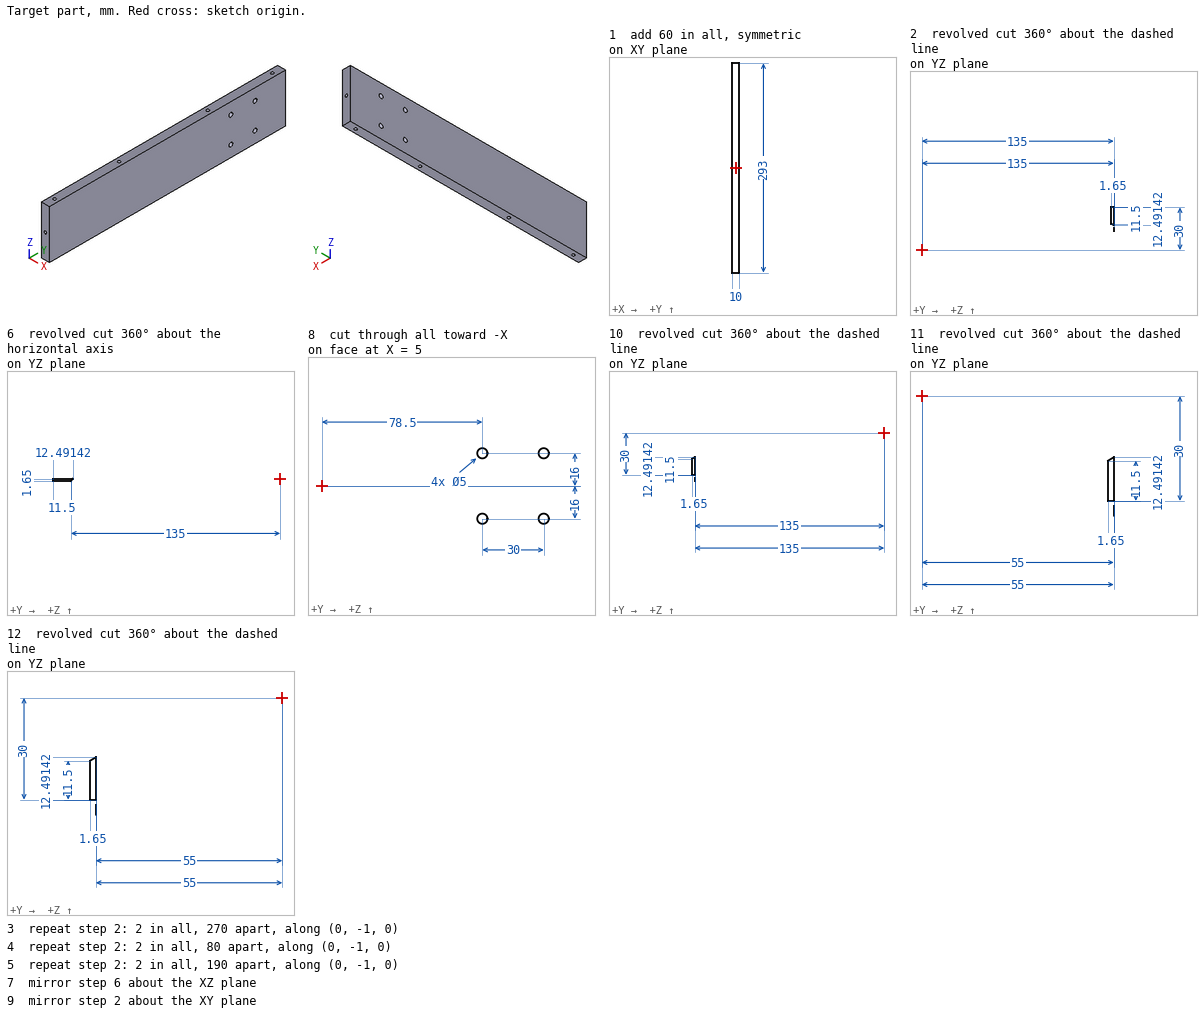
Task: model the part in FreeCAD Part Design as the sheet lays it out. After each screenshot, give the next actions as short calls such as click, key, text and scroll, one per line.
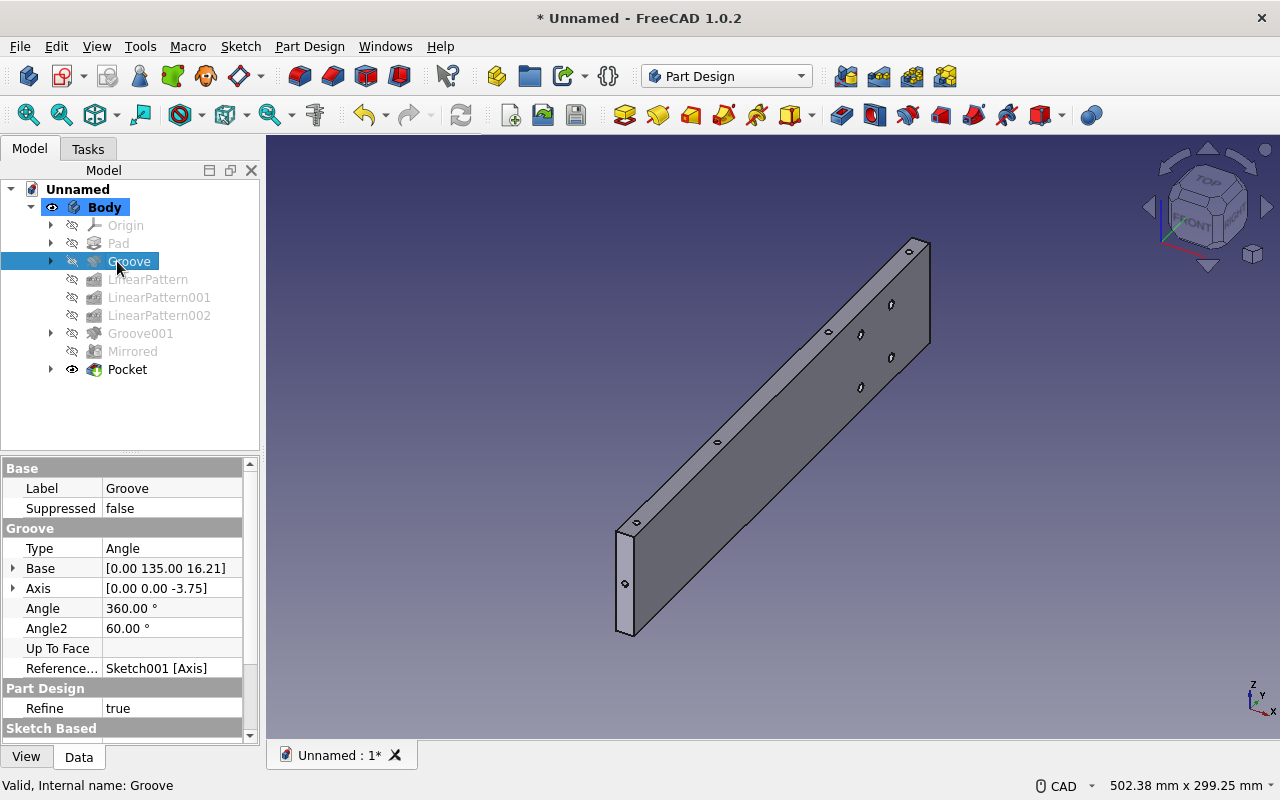
click(846, 76)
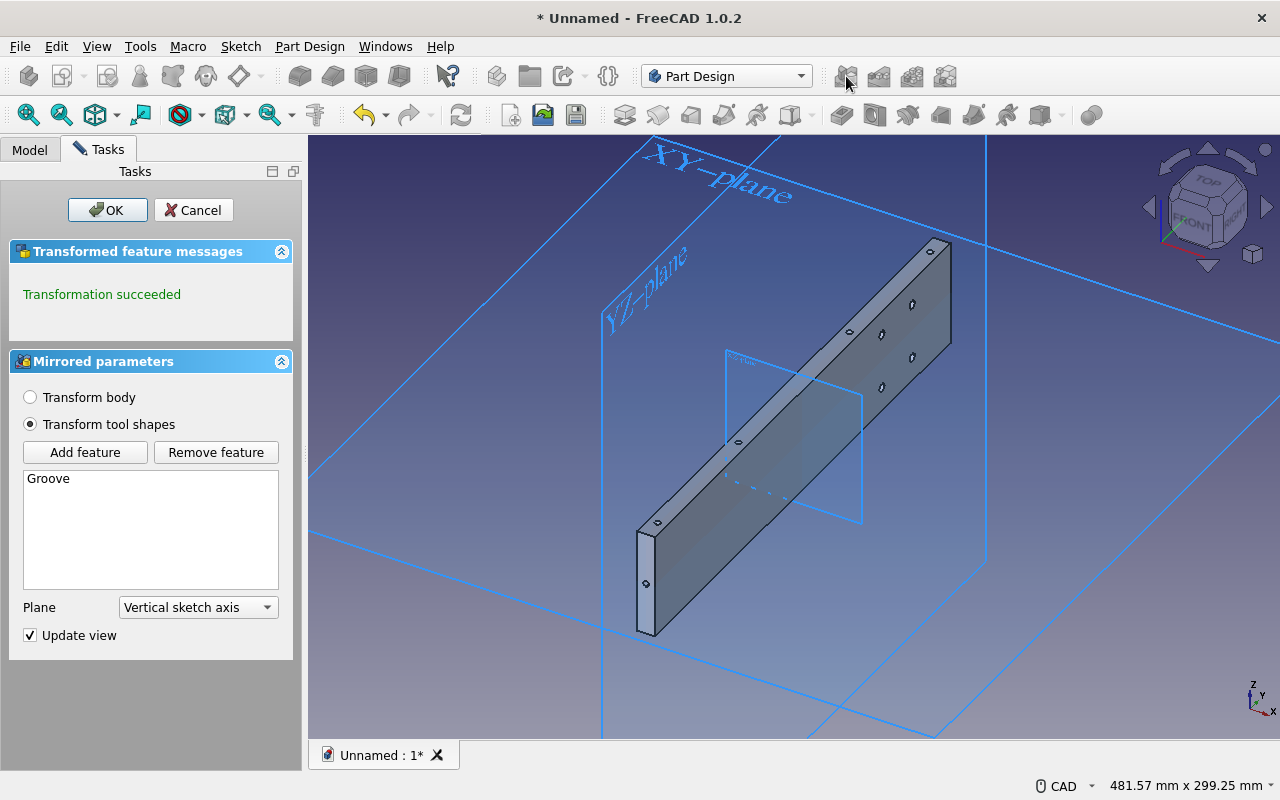
click(199, 608)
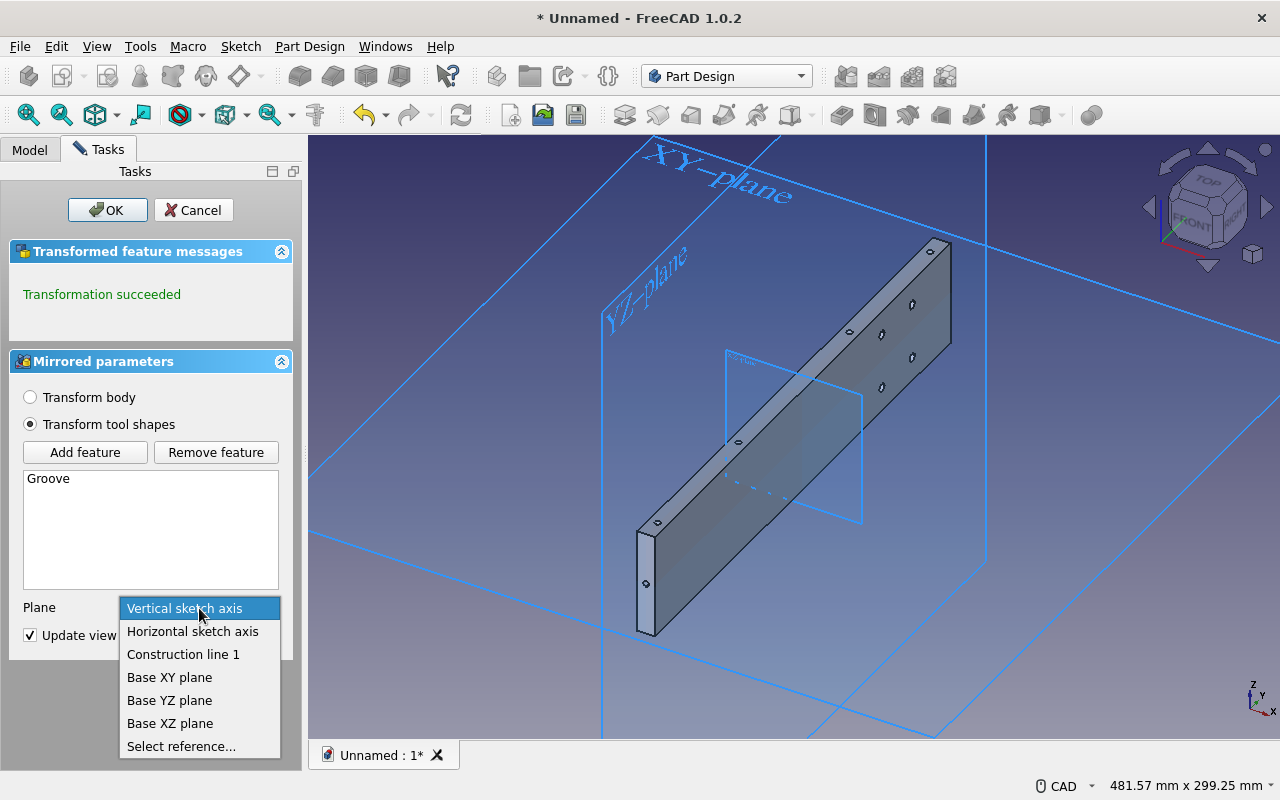
click(198, 678)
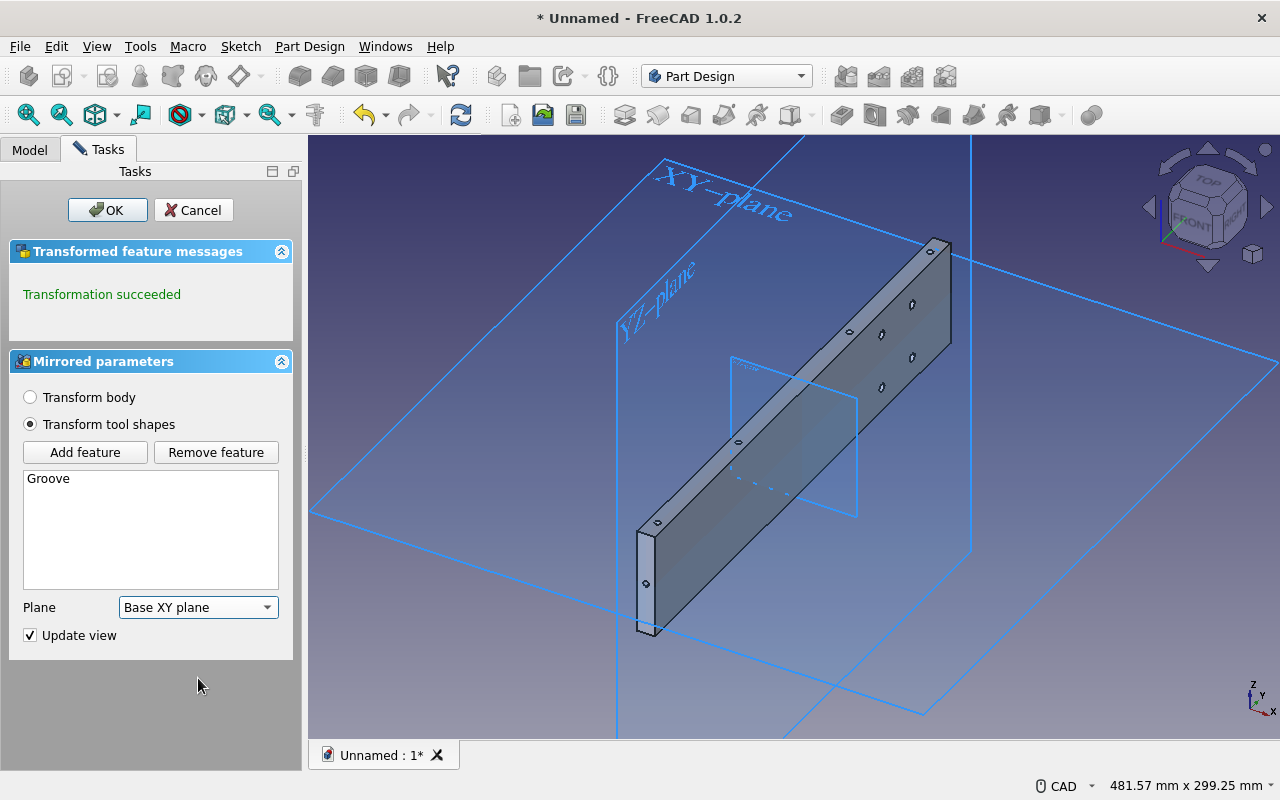
click(108, 210)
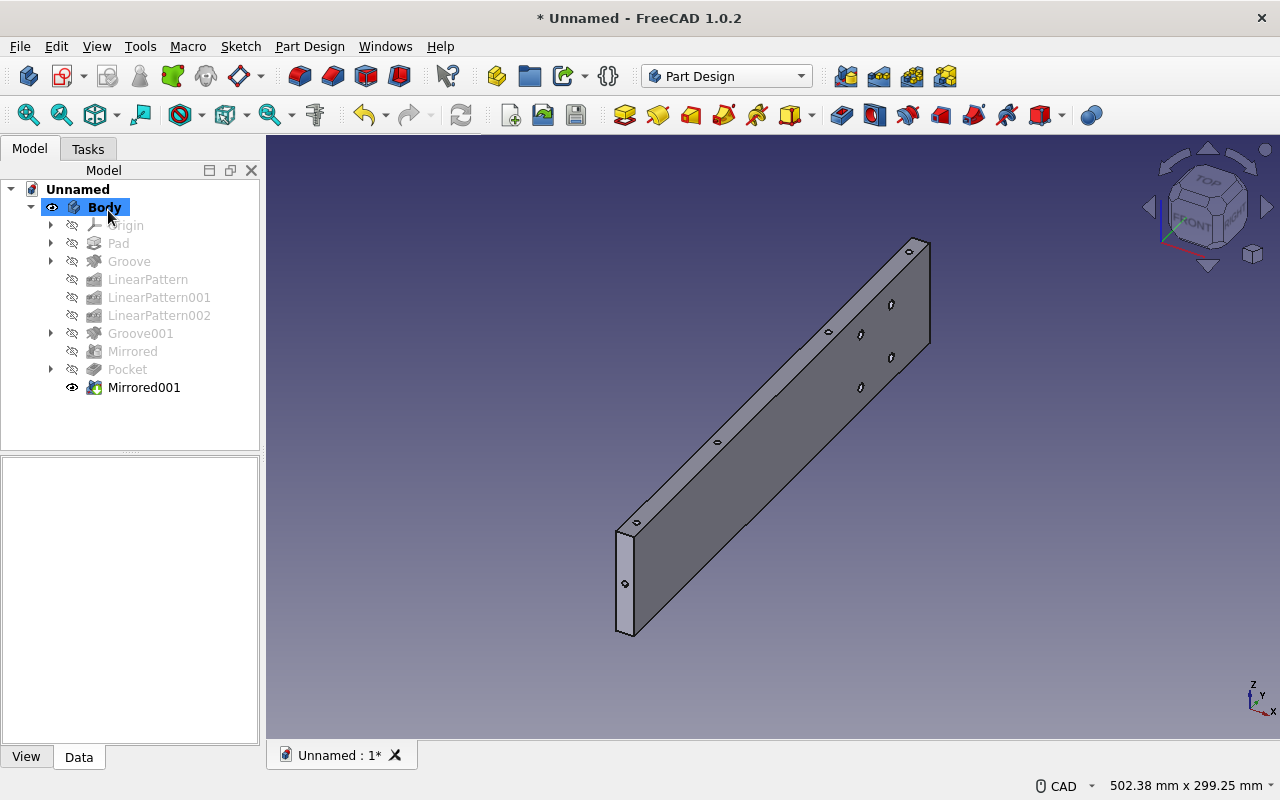
click(62, 76)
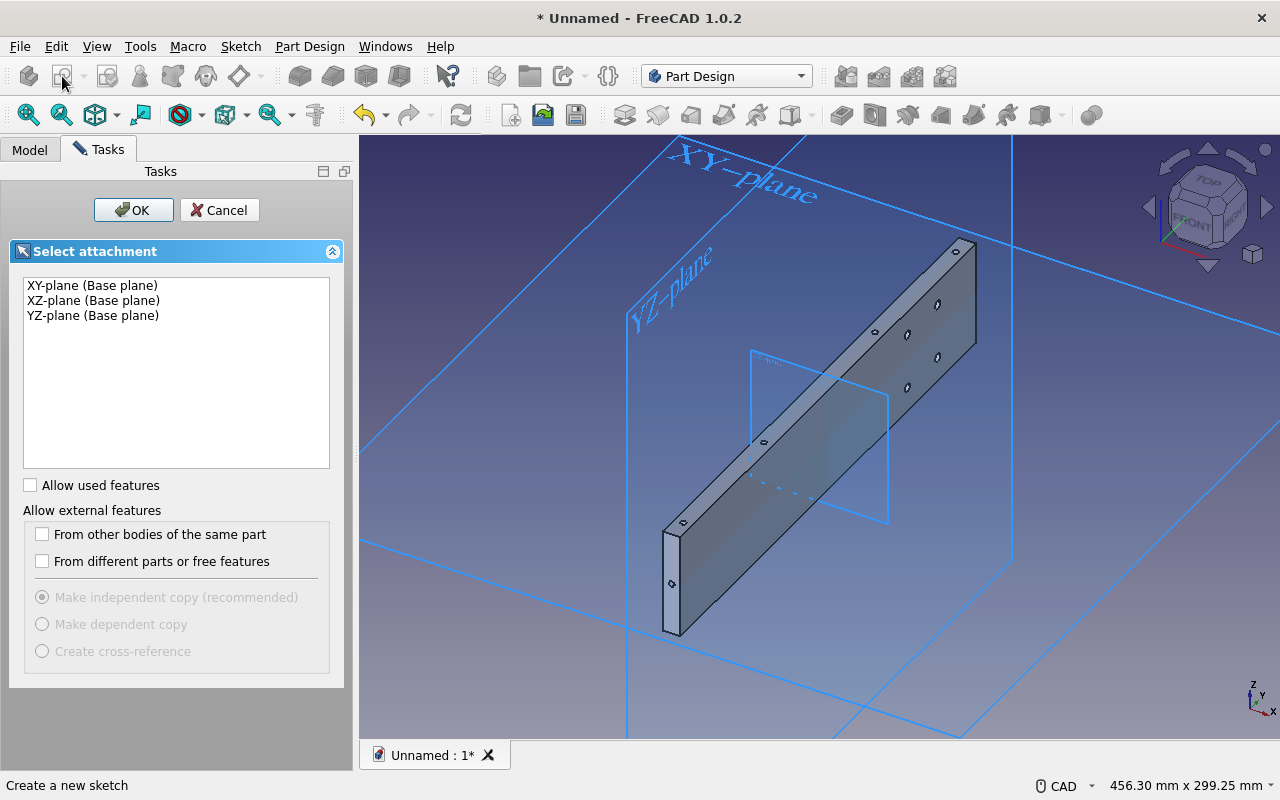
click(84, 316)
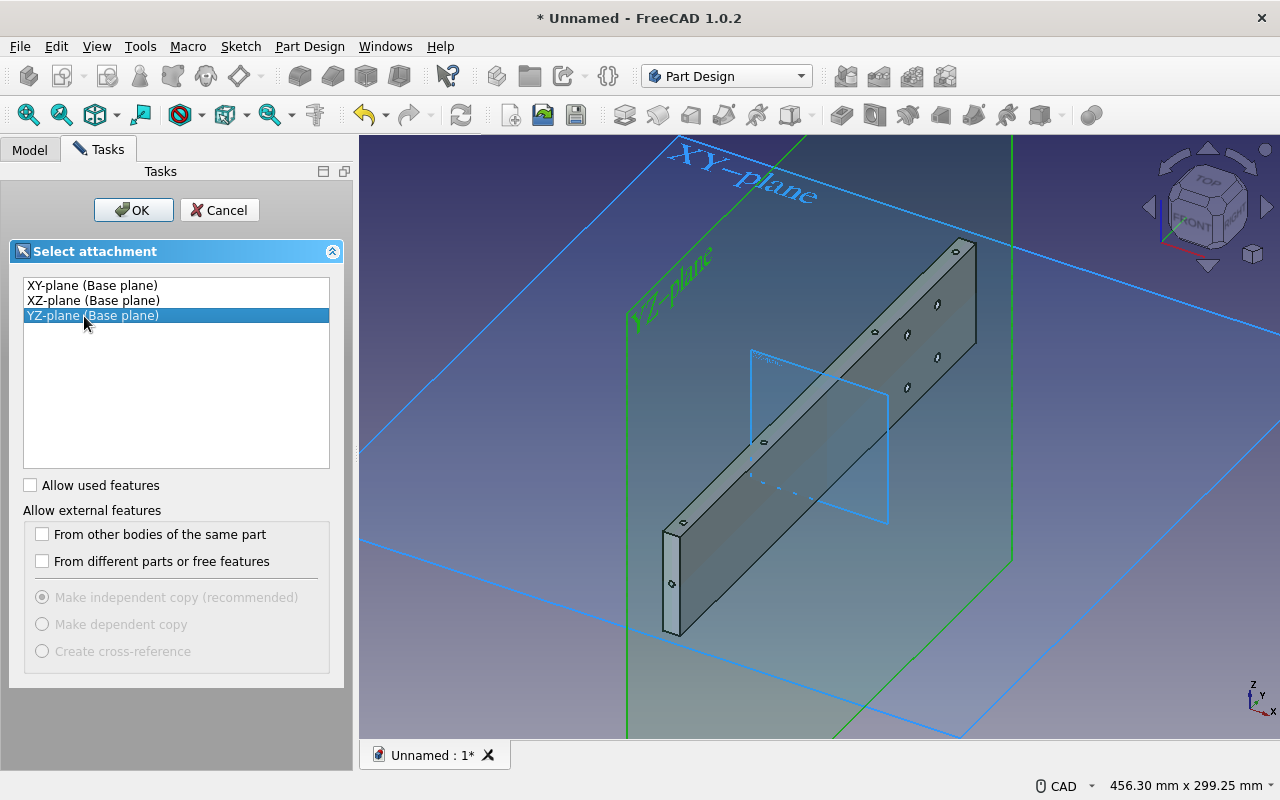
click(134, 210)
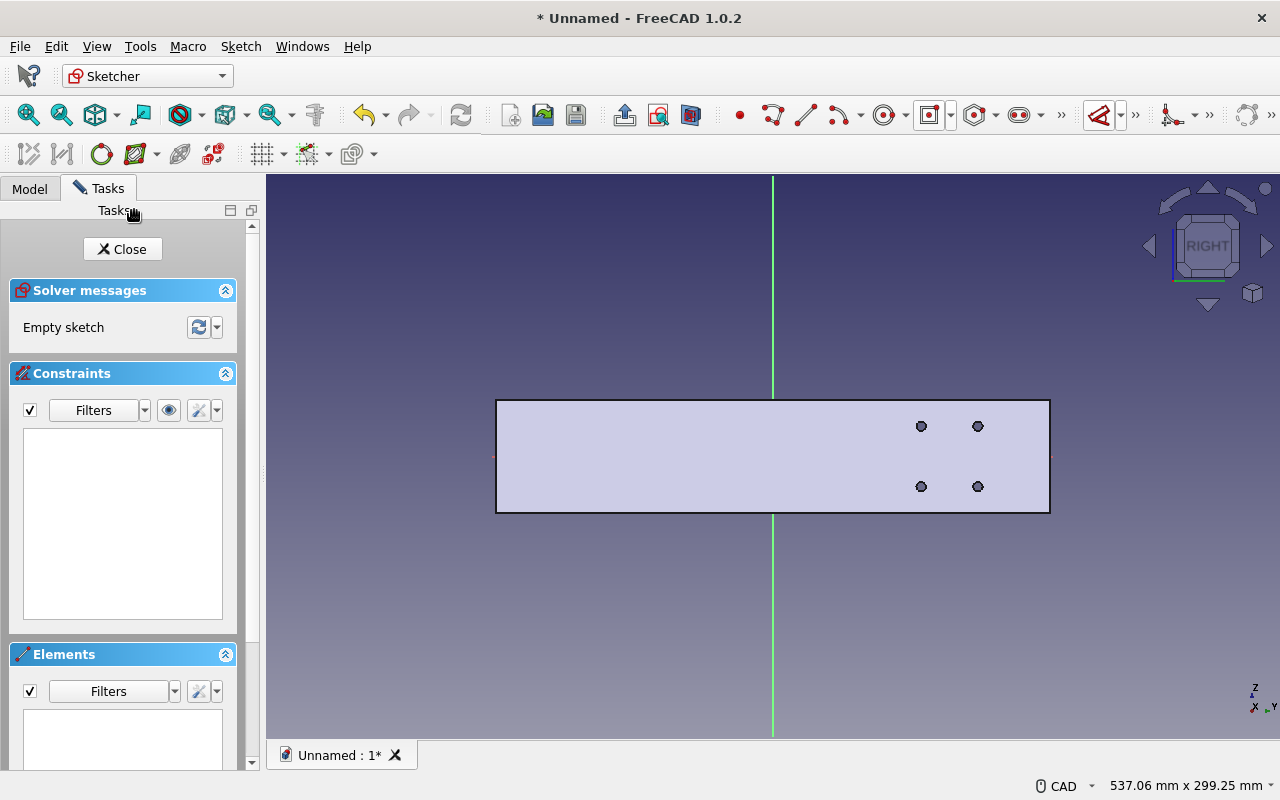
click(691, 116)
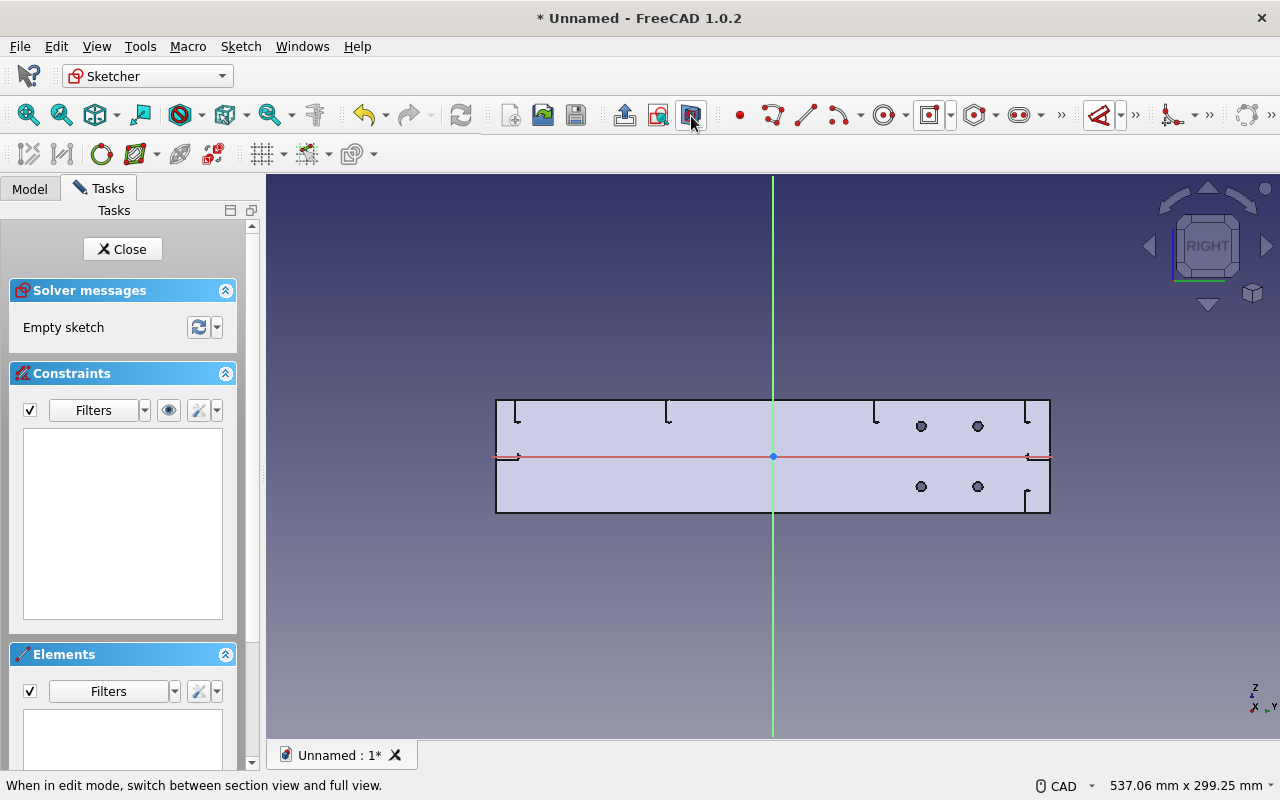
scroll(498, 511, up, 12)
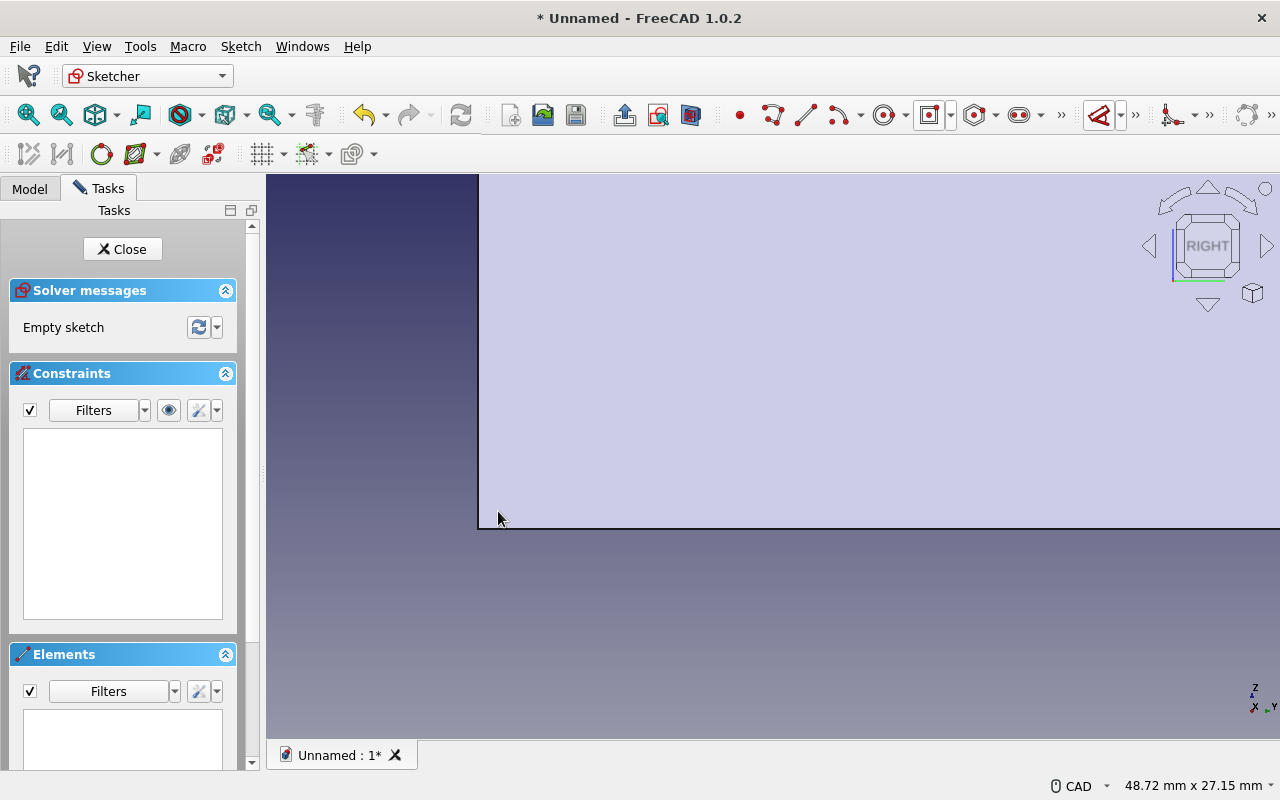
click(773, 116)